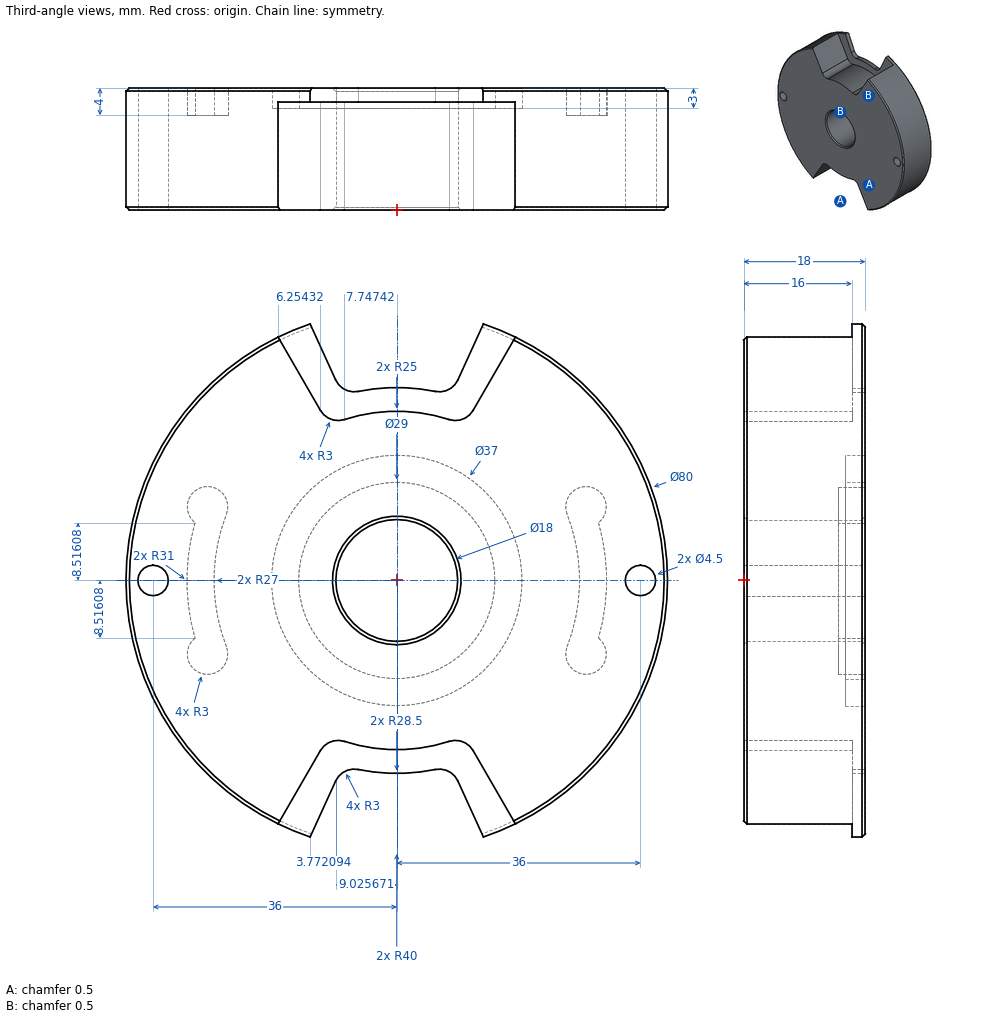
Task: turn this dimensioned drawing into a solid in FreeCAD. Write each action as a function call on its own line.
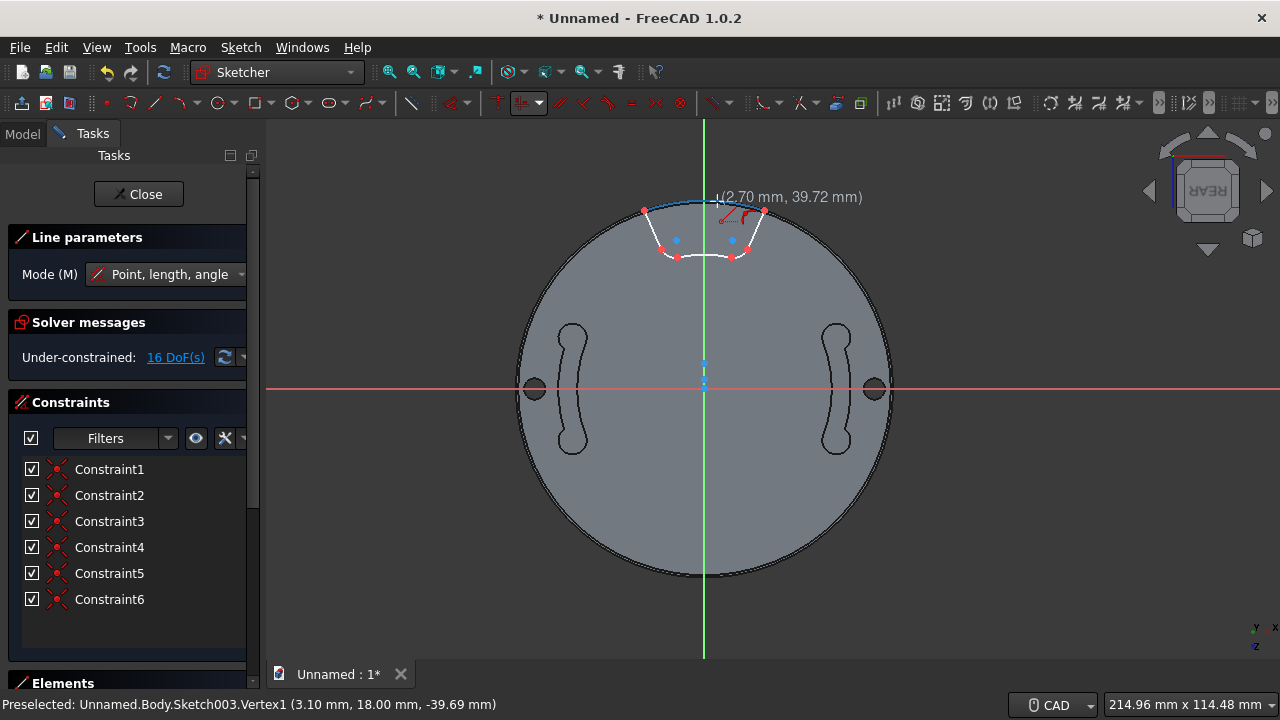
click(765, 568)
click(747, 529)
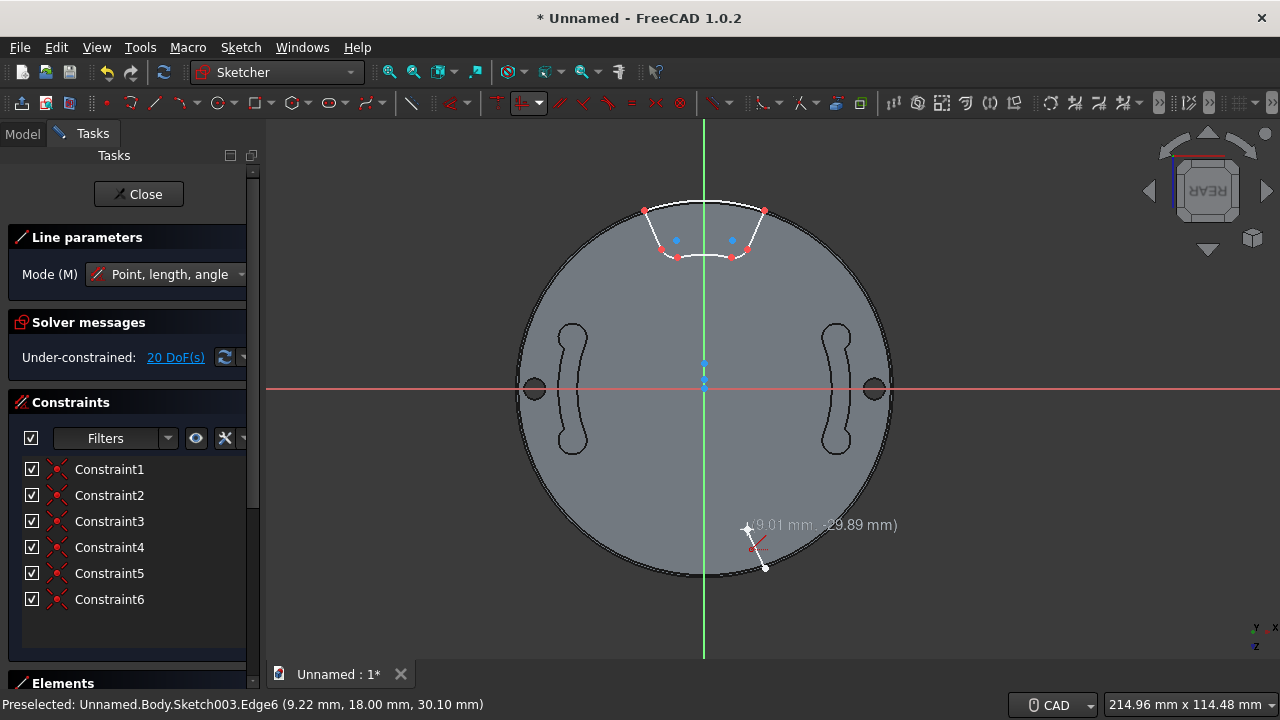
click(662, 529)
click(644, 568)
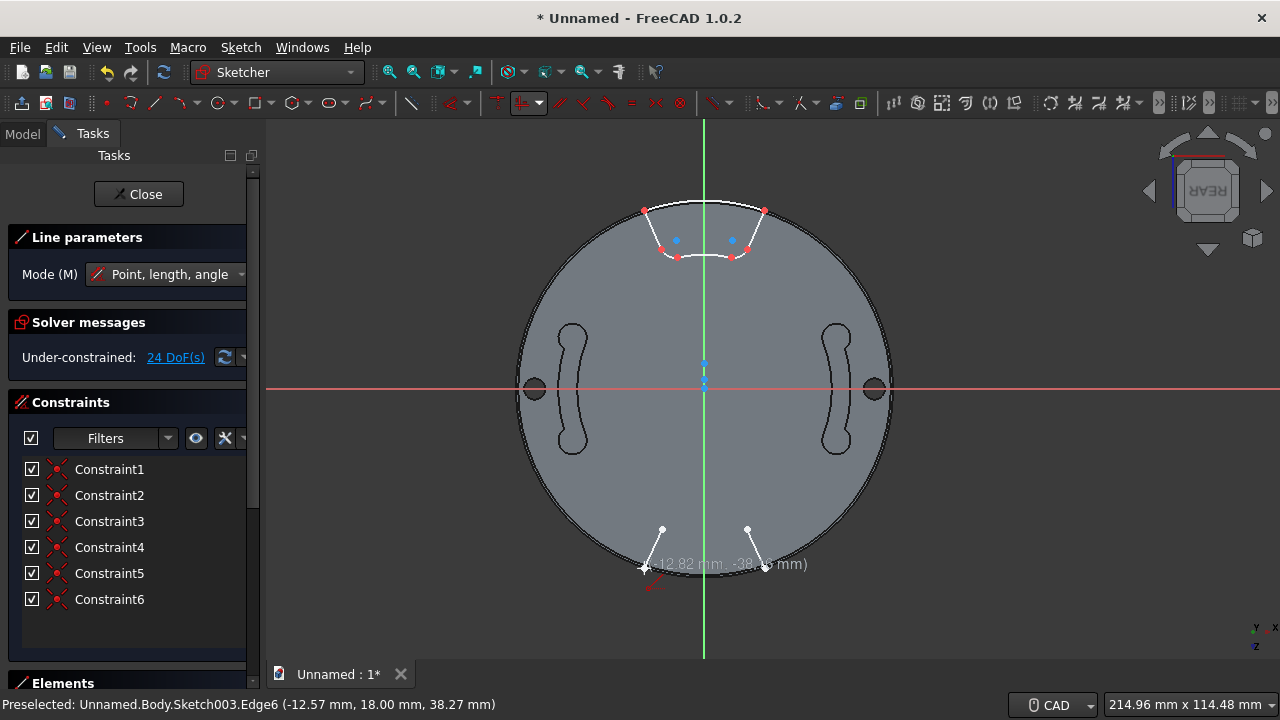
click(180, 104)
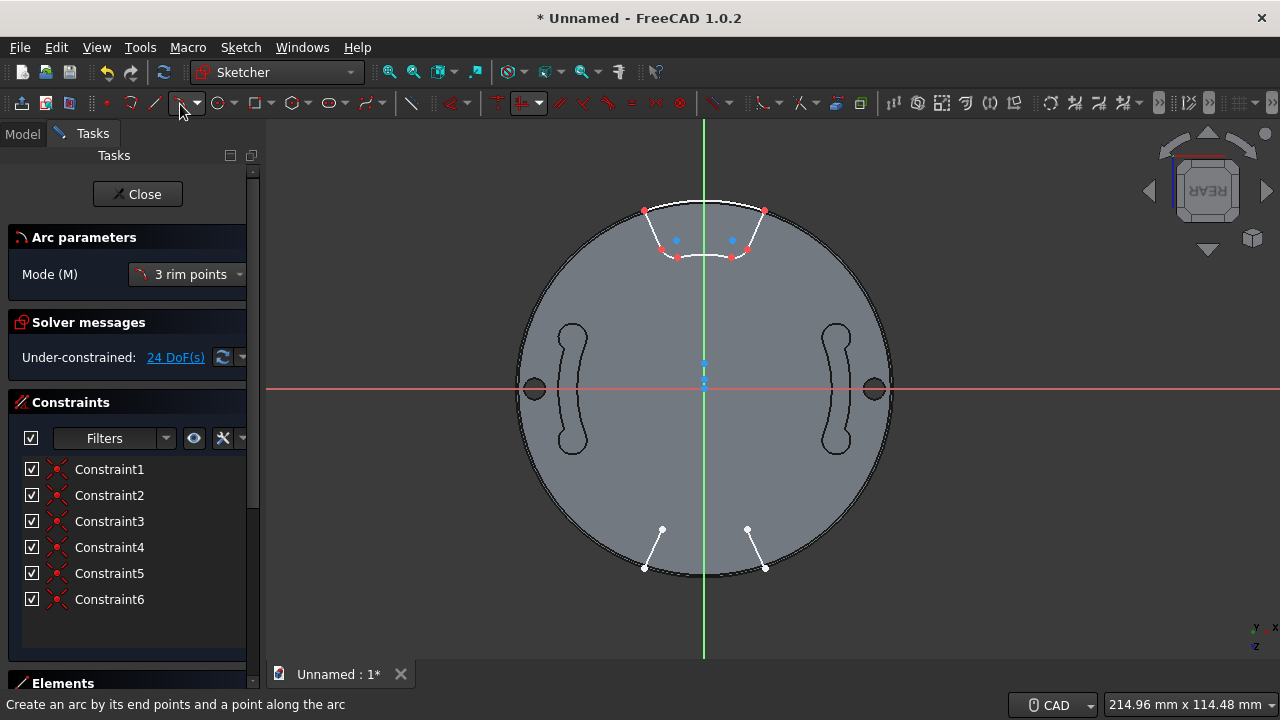
click(747, 530)
click(731, 521)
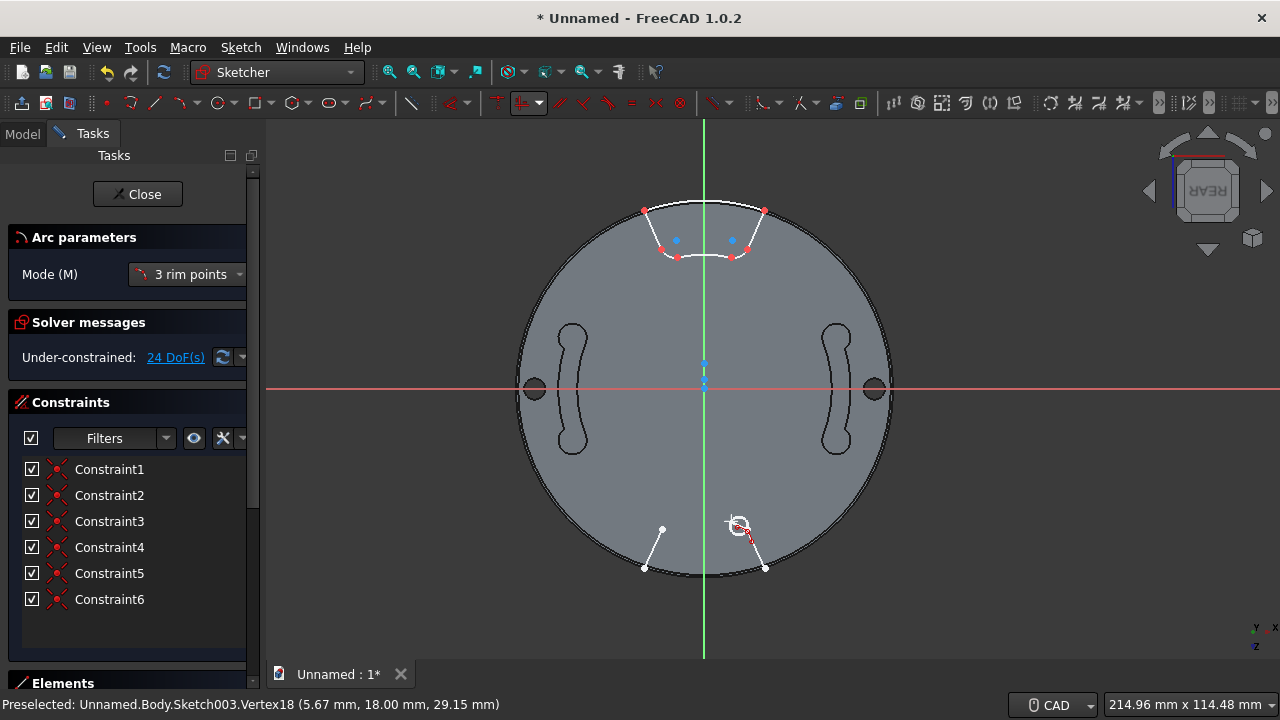
scroll(741, 522, up, 9)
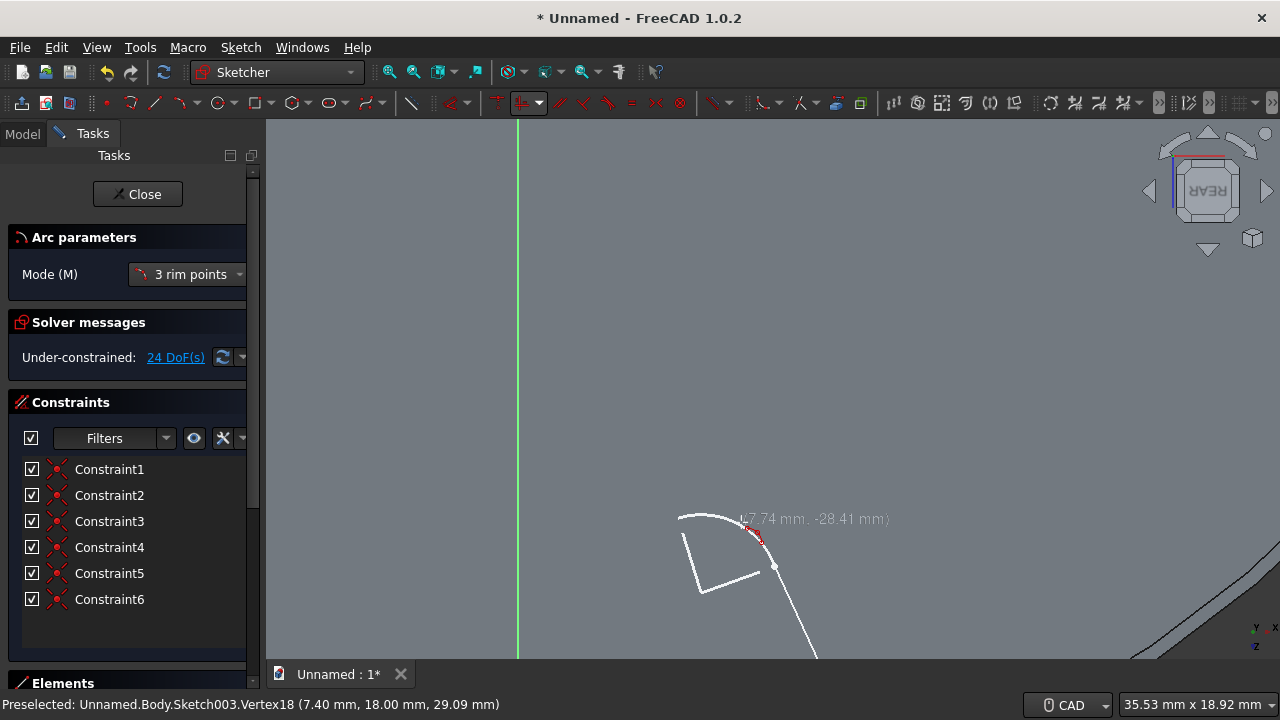
click(736, 518)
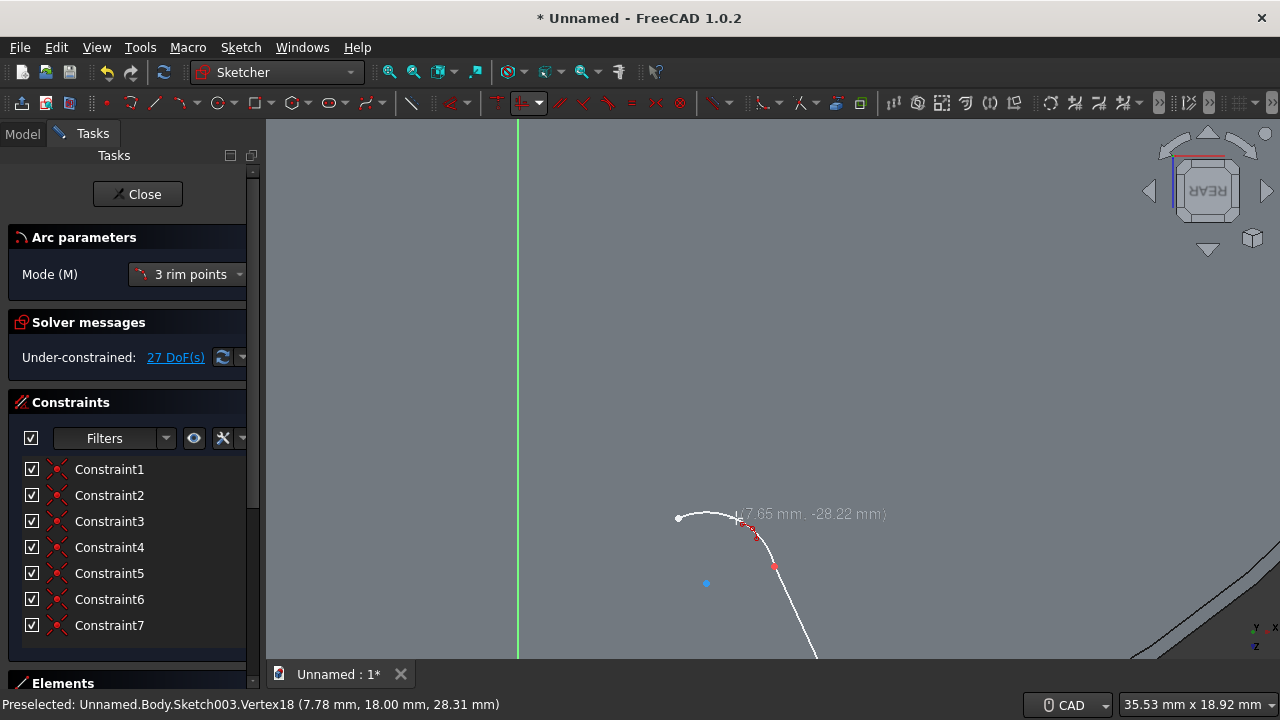
scroll(741, 523, down, 9)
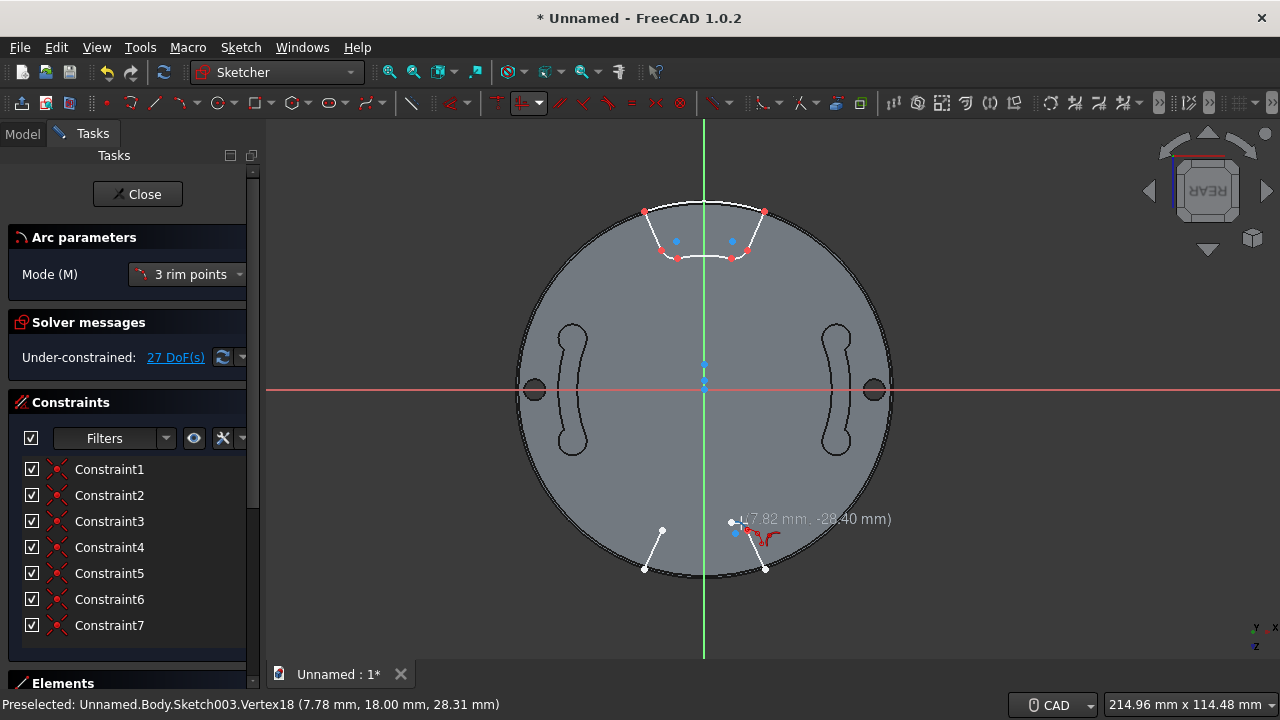
click(731, 523)
click(678, 522)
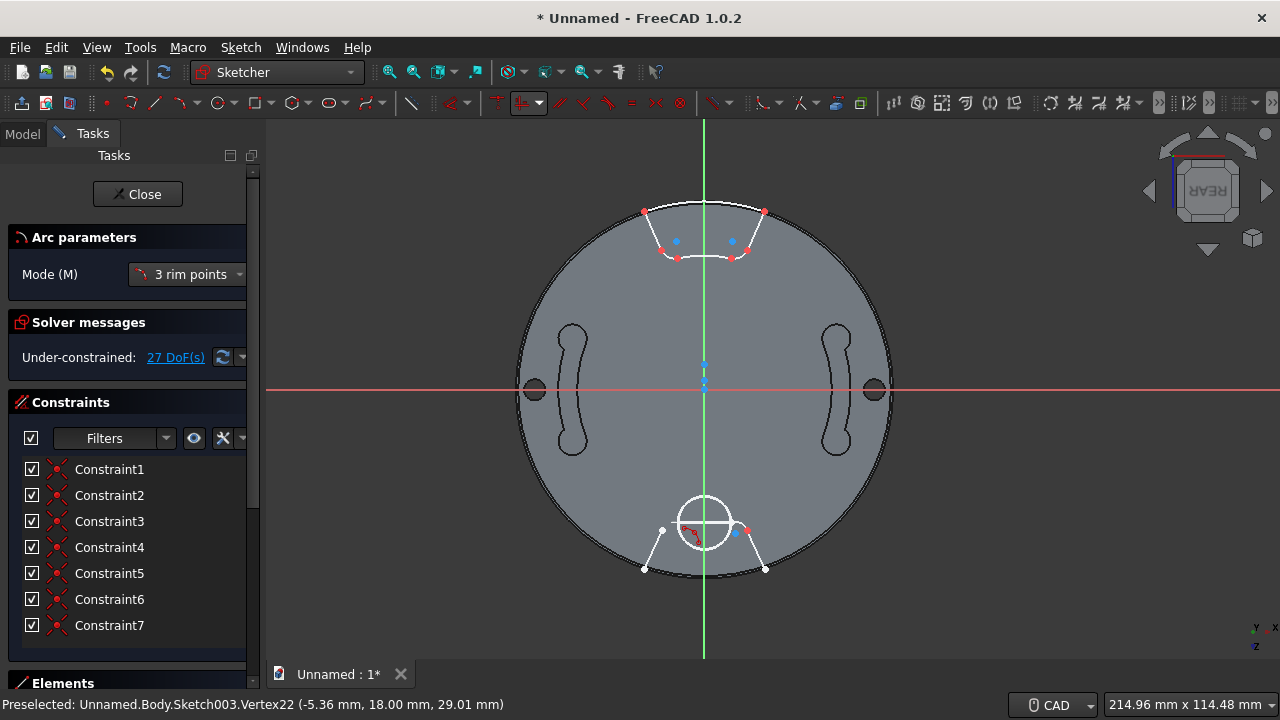
scroll(699, 524, up, 10)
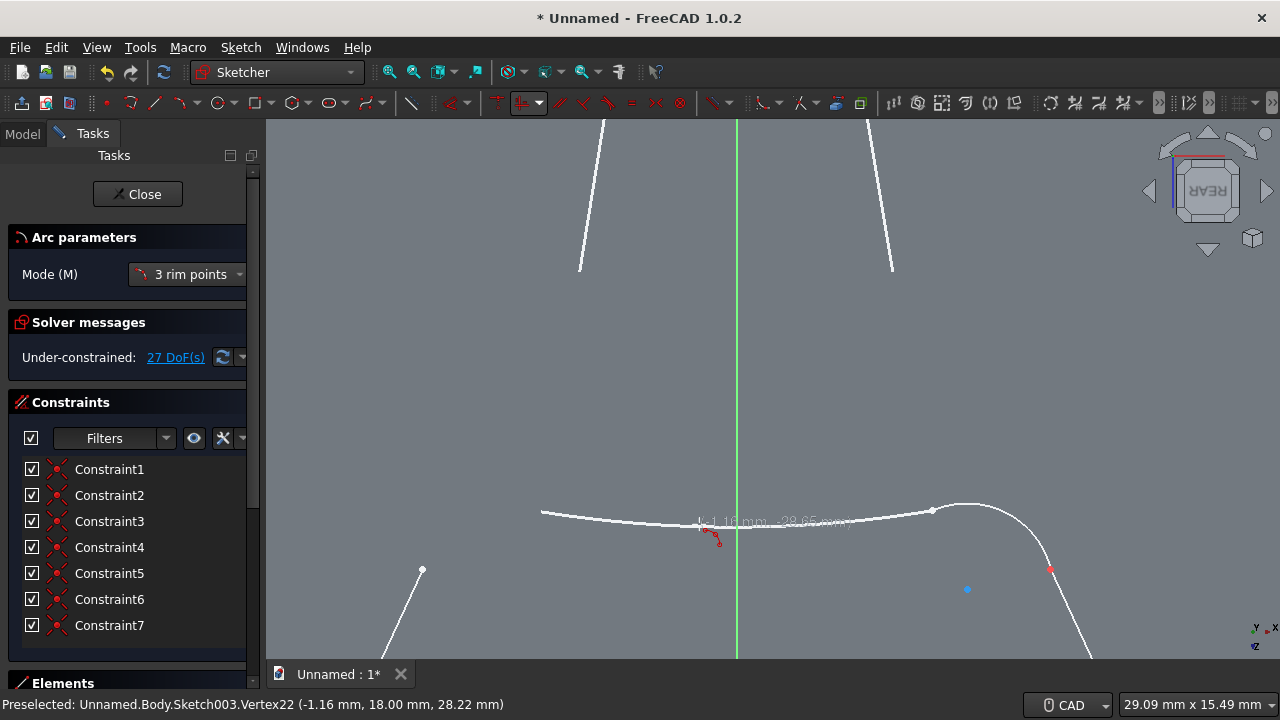
click(697, 520)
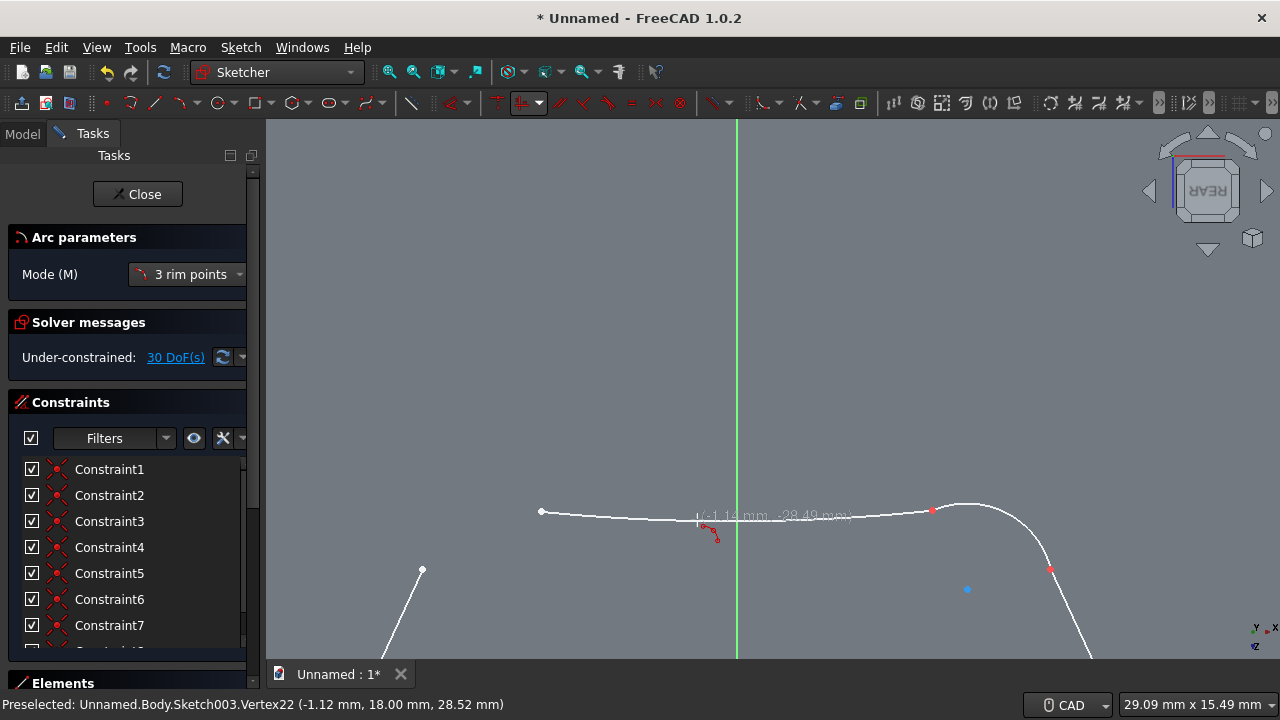
scroll(699, 524, down, 10)